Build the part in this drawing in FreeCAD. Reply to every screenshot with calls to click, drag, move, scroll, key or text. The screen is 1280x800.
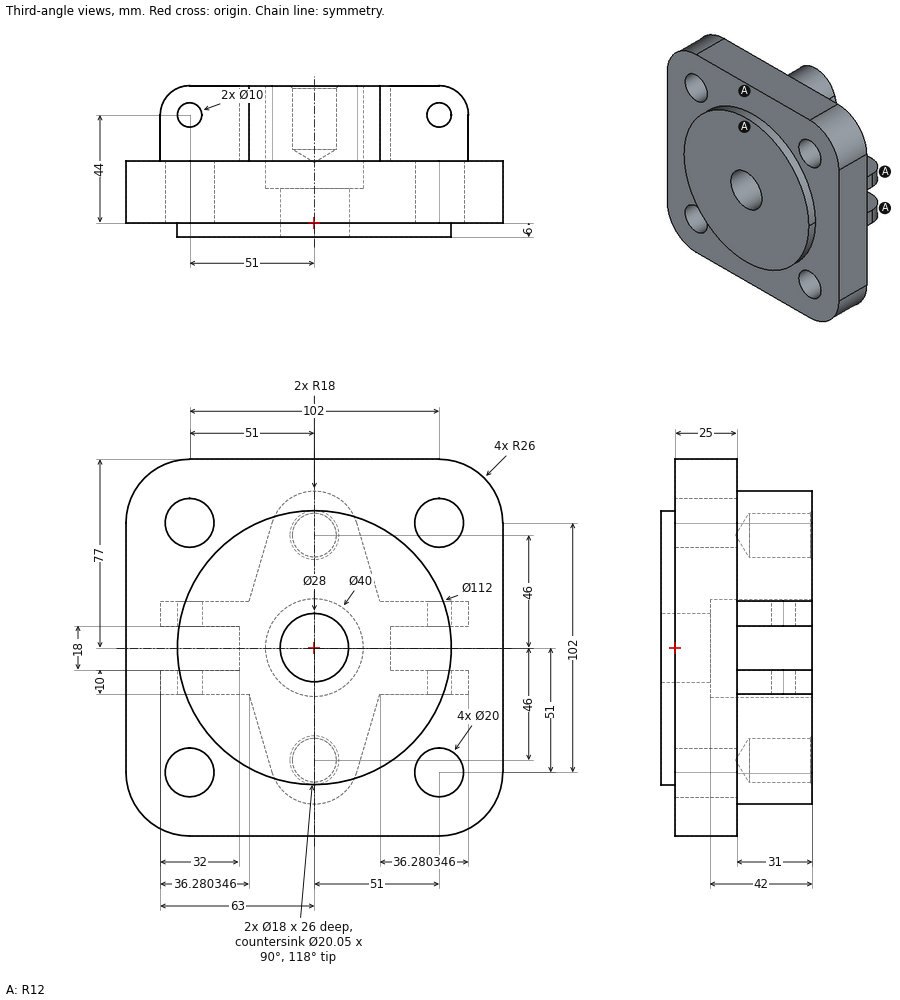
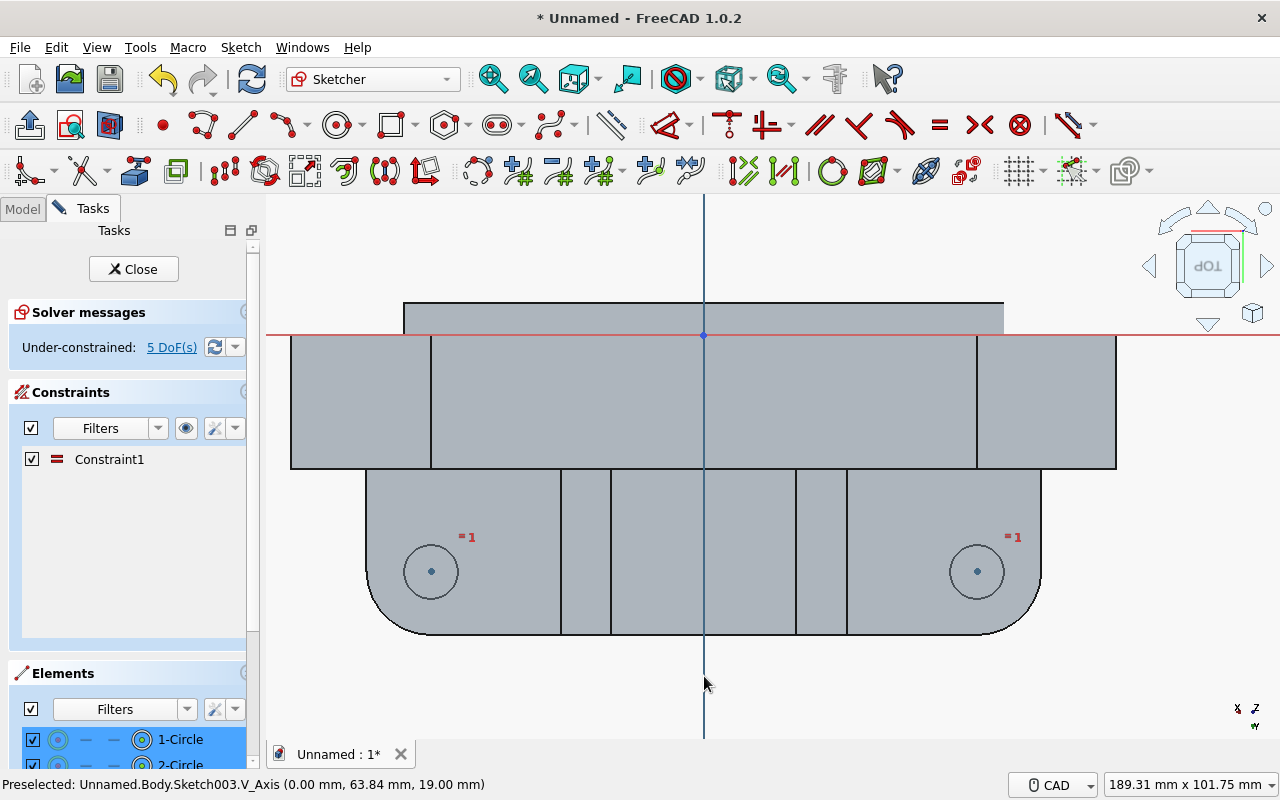
key(s)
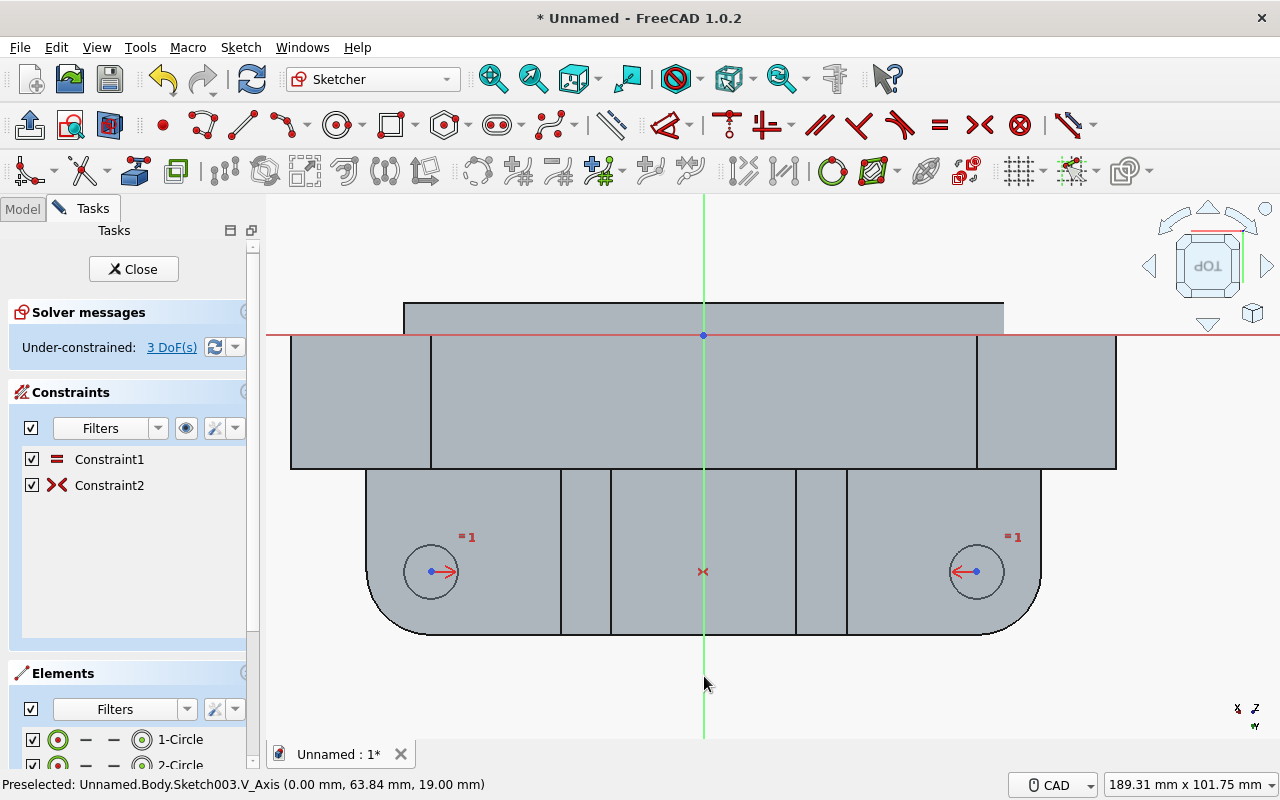
key(d)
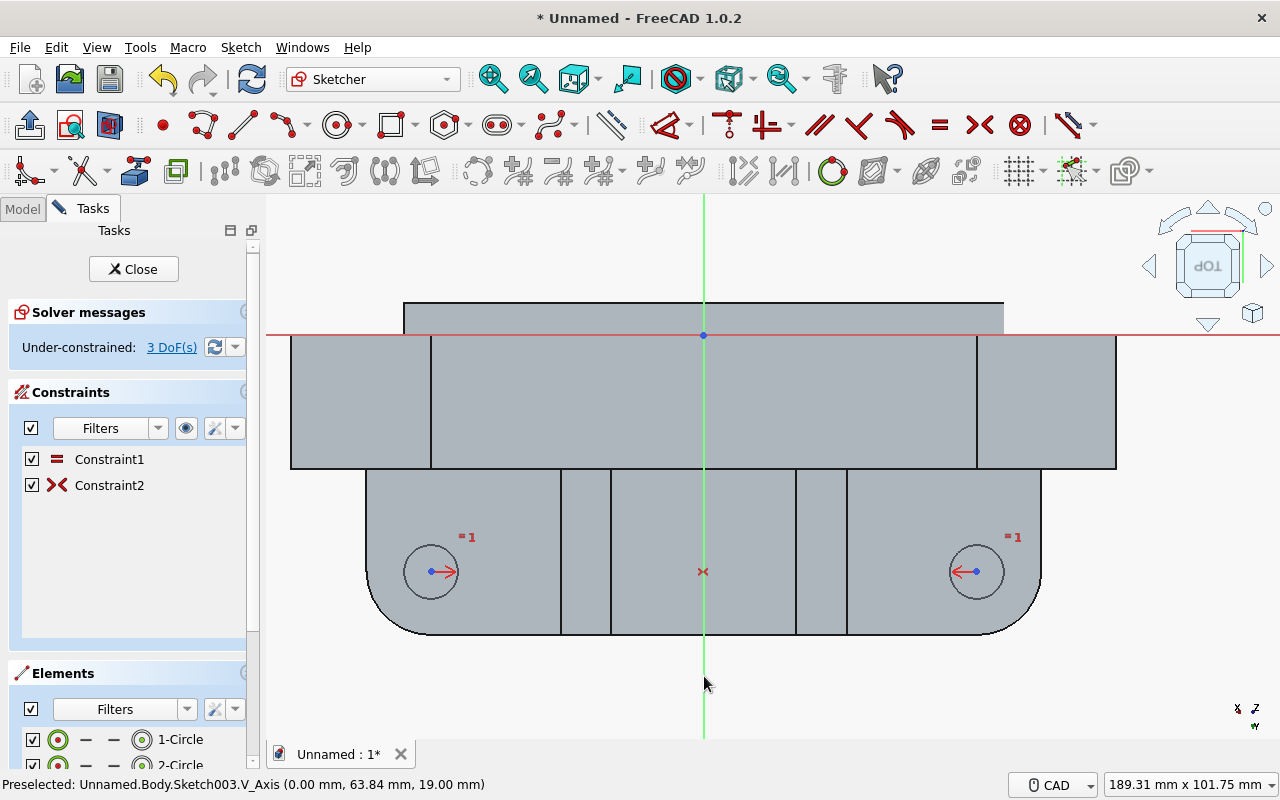
click(996, 553)
click(1019, 530)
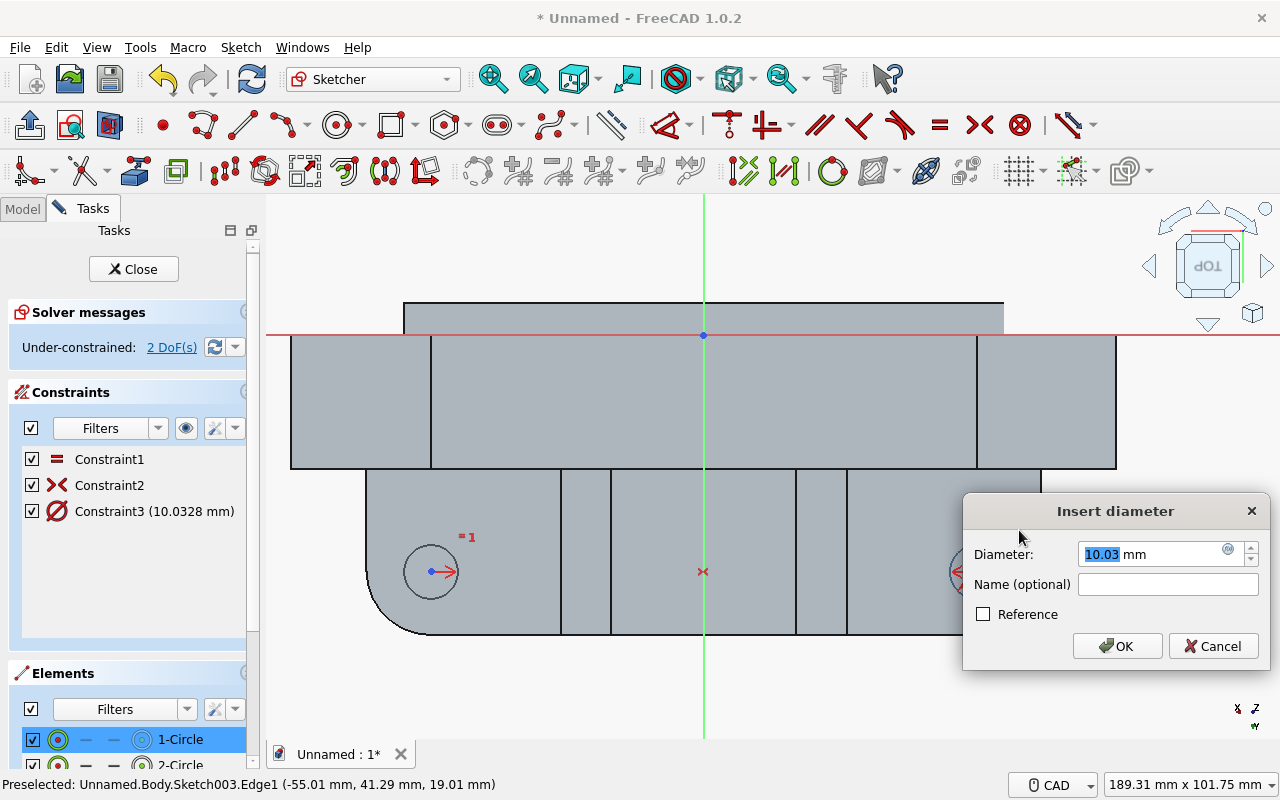
text(10)
key(Return)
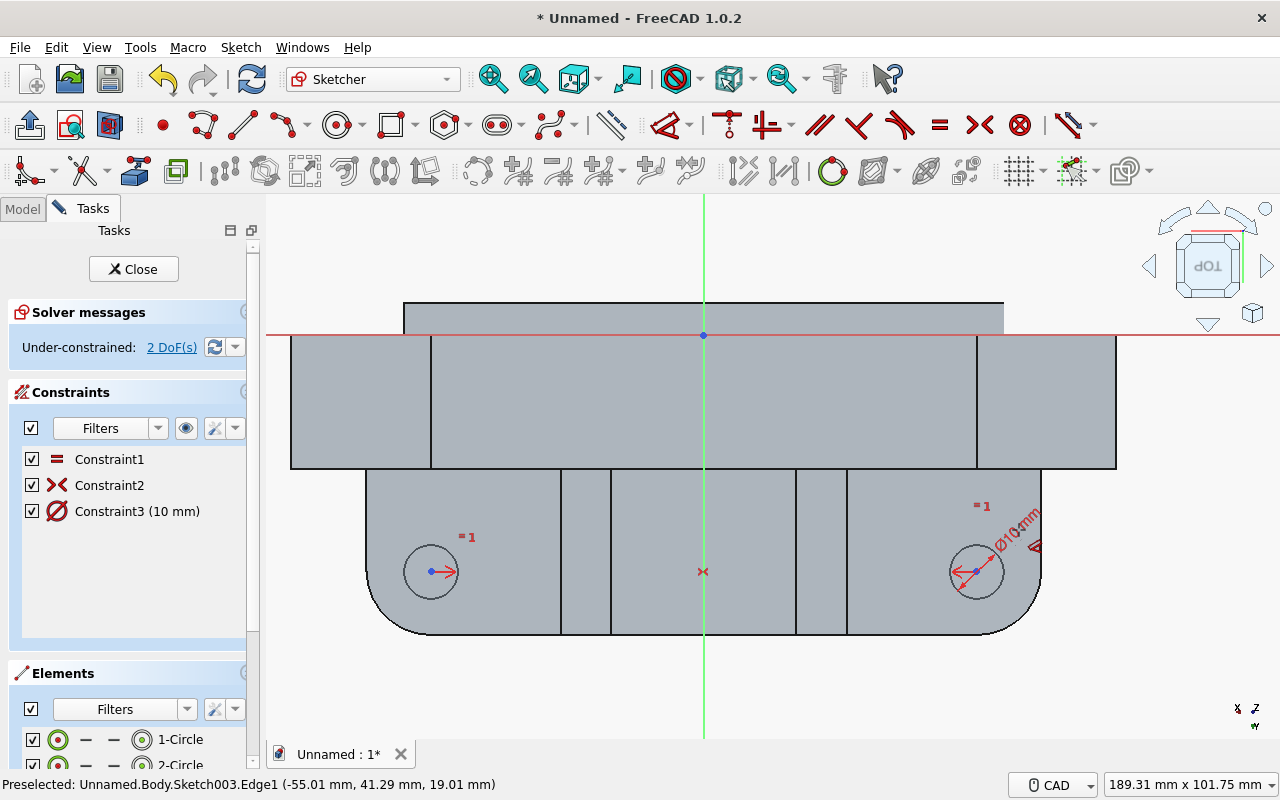
click(977, 572)
click(840, 301)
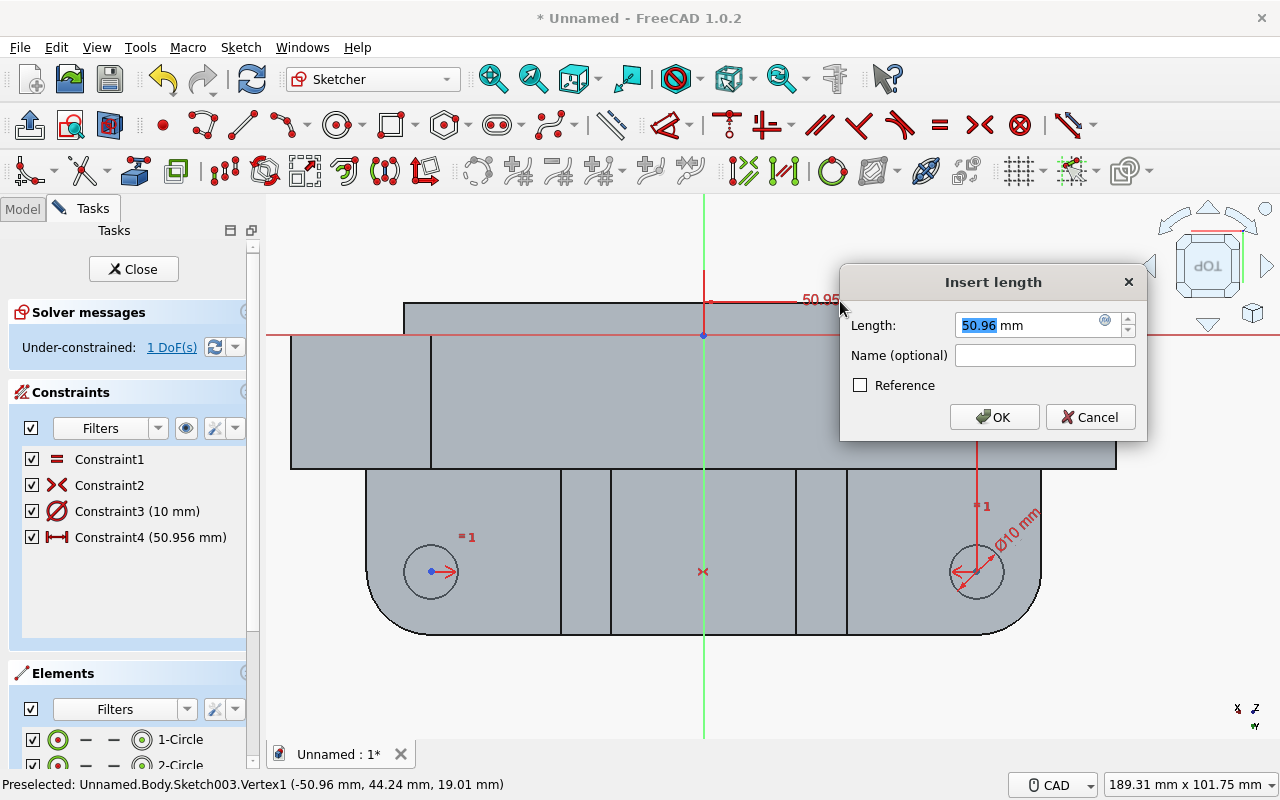
text(51)
key(Return)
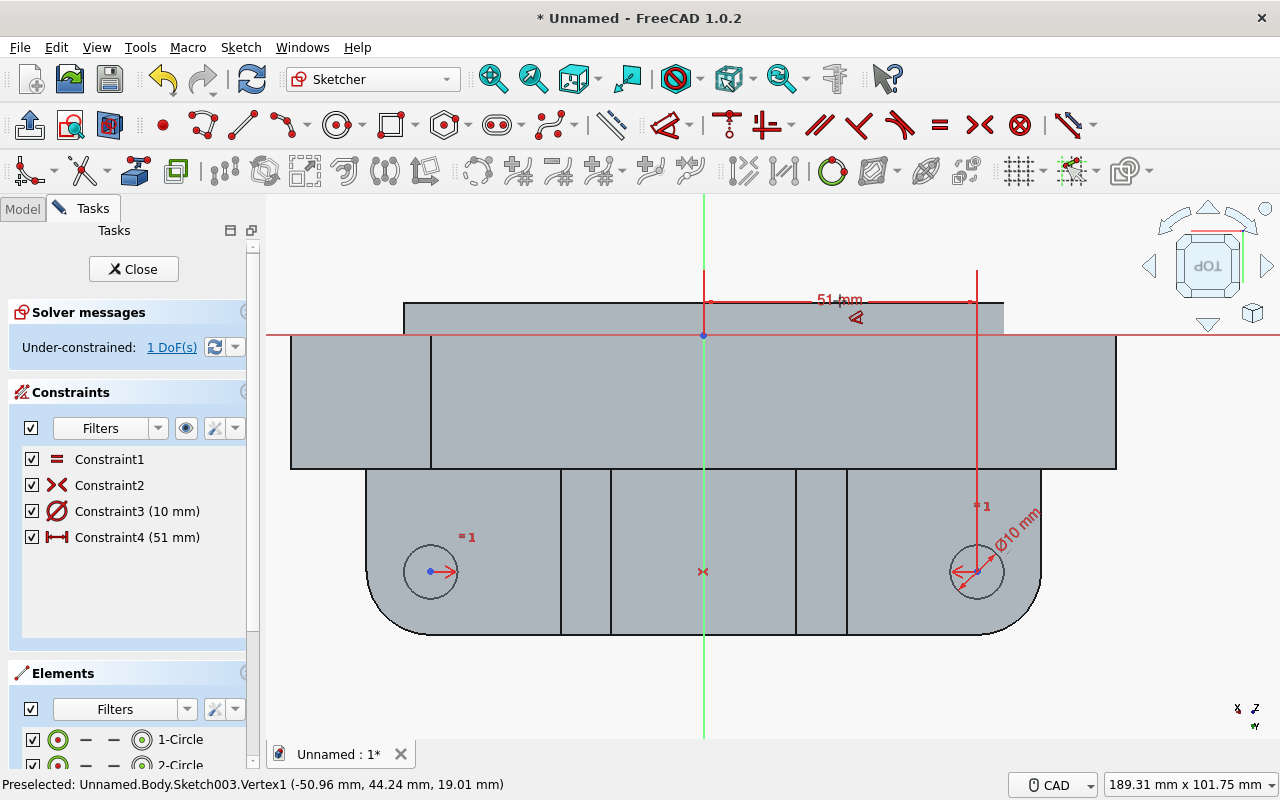
click(977, 572)
click(1011, 454)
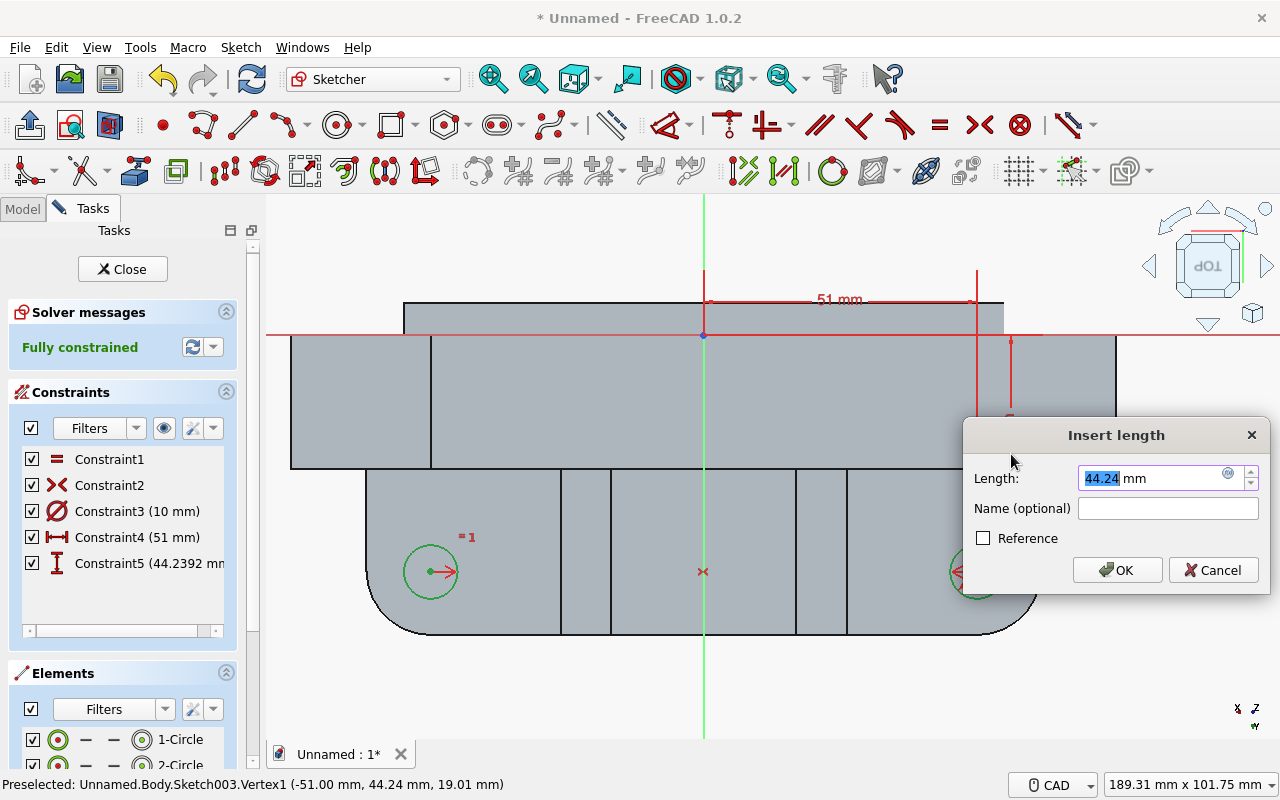
text(44)
key(Return)
key(Escape)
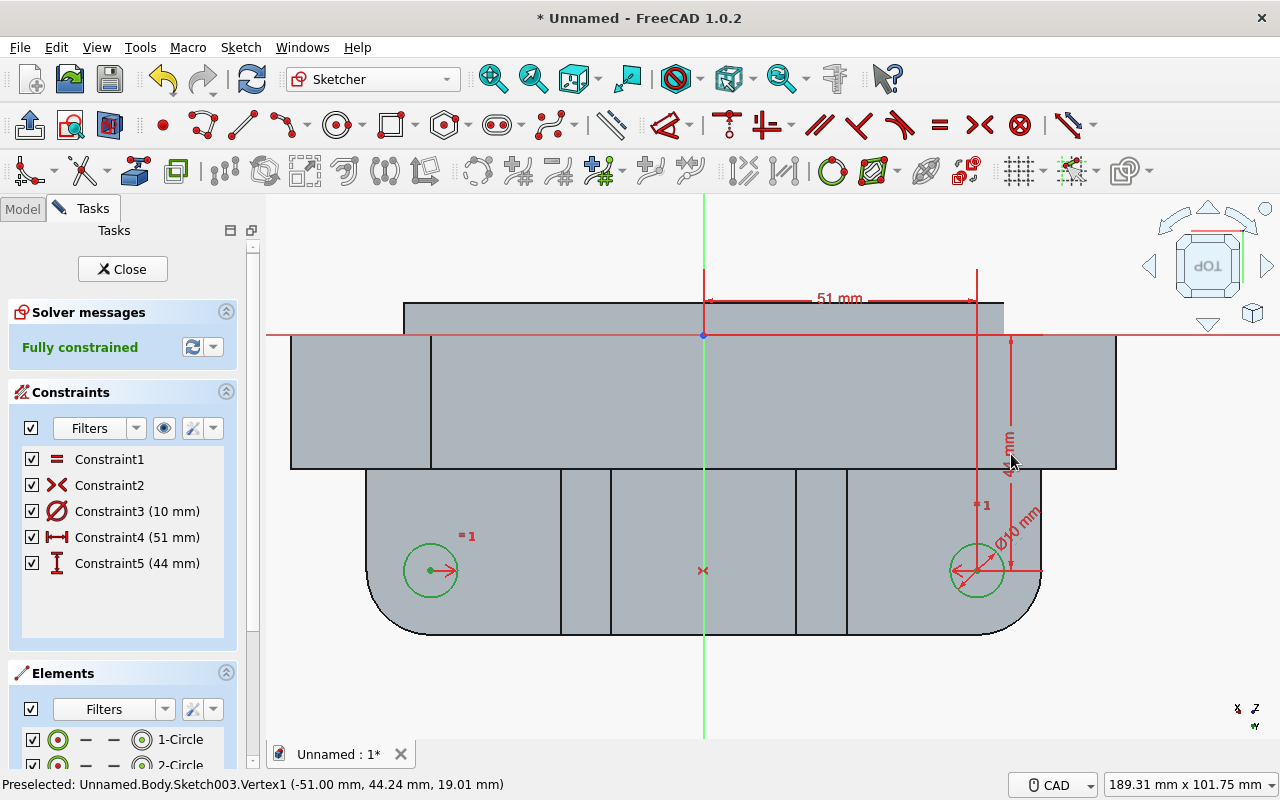
click(123, 269)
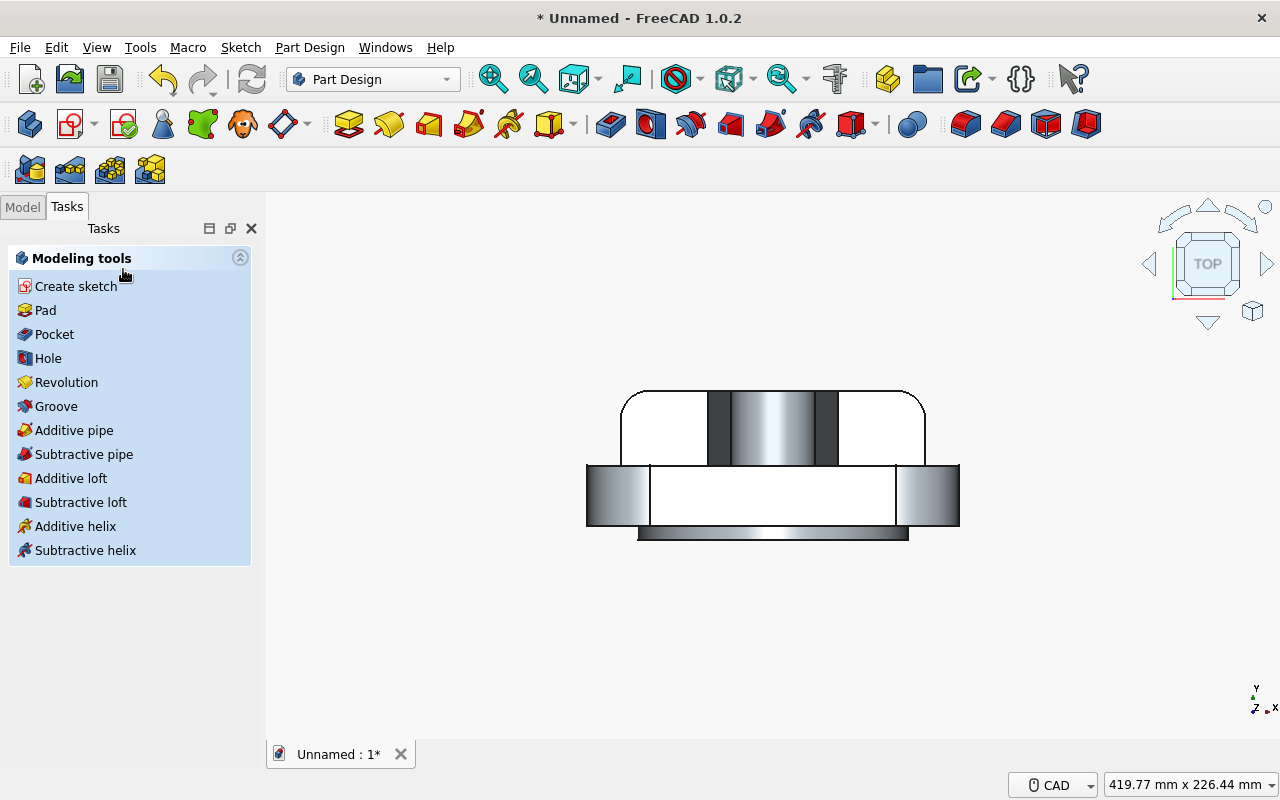
click(612, 124)